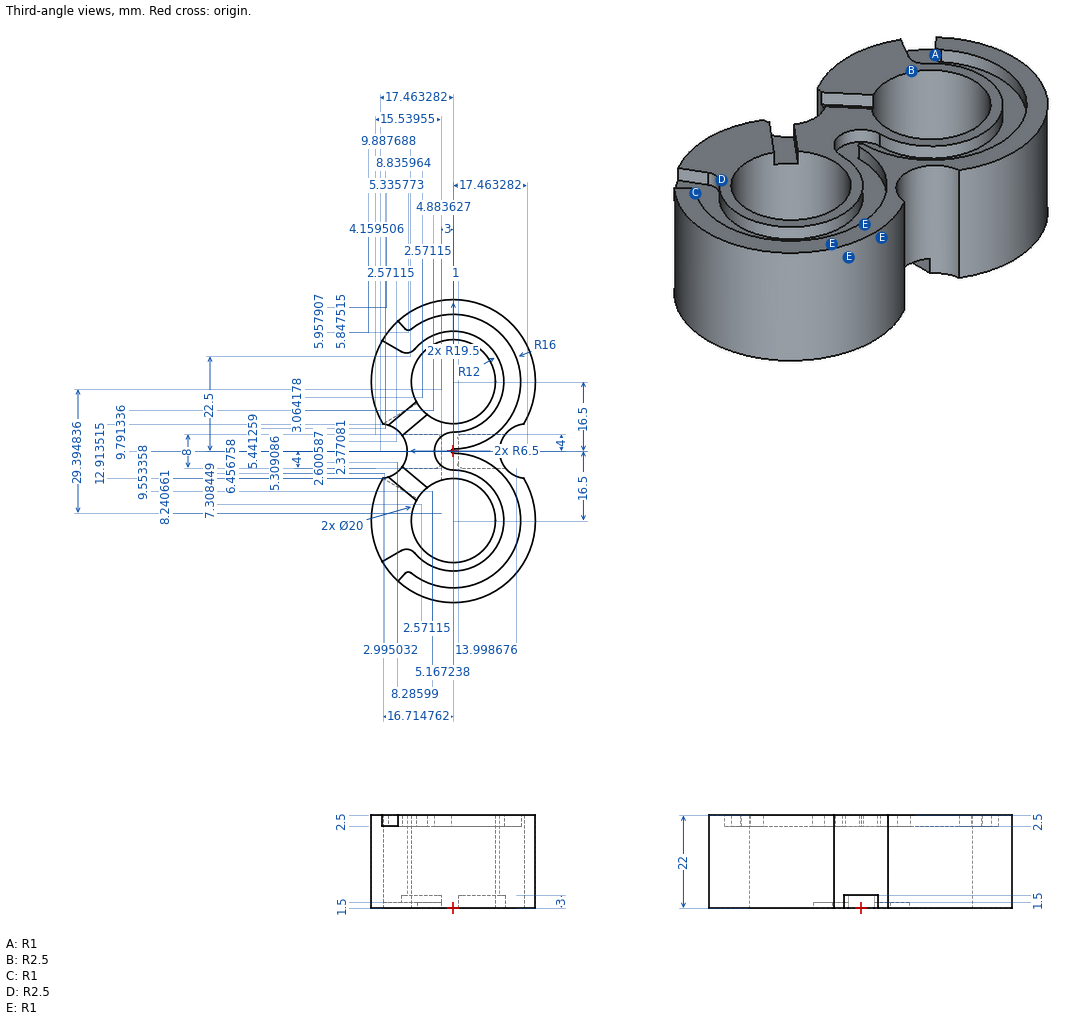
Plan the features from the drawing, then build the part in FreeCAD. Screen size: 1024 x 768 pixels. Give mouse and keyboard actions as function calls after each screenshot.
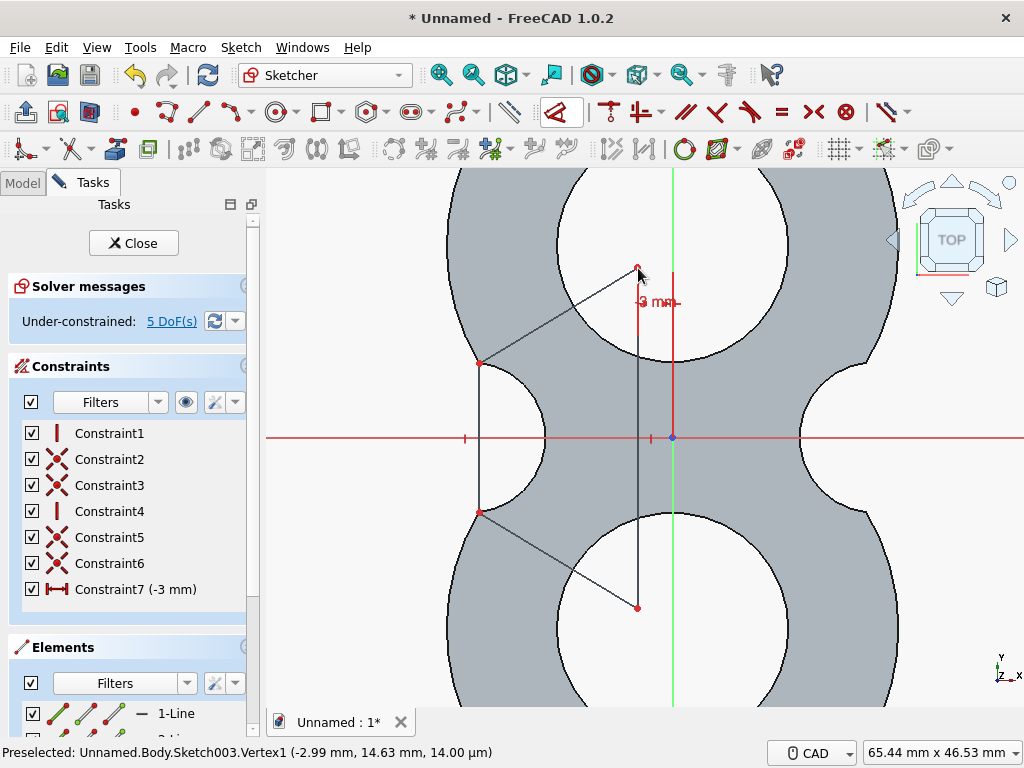
click(638, 370)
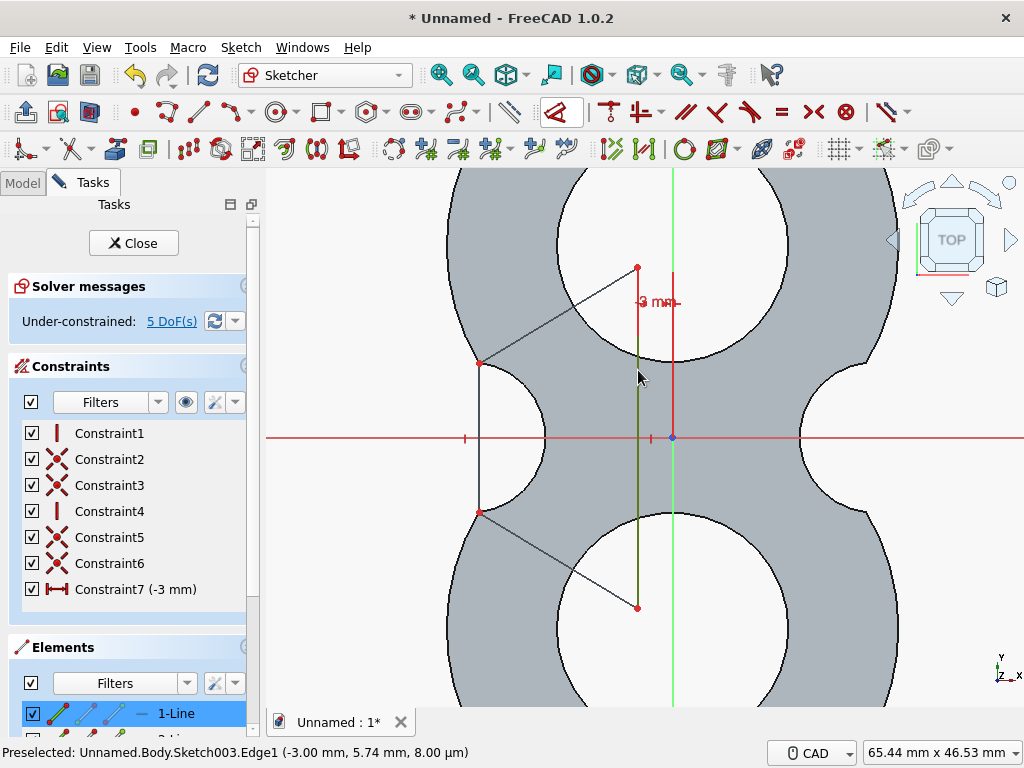
key(i)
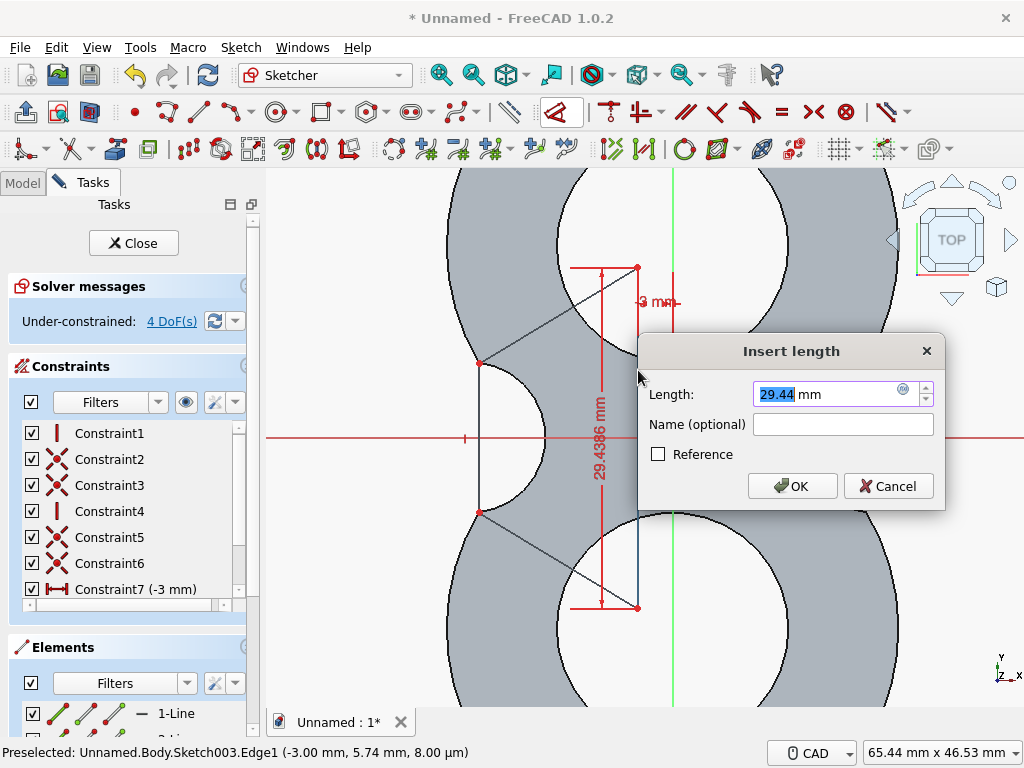
text(29.394836)
key(Return)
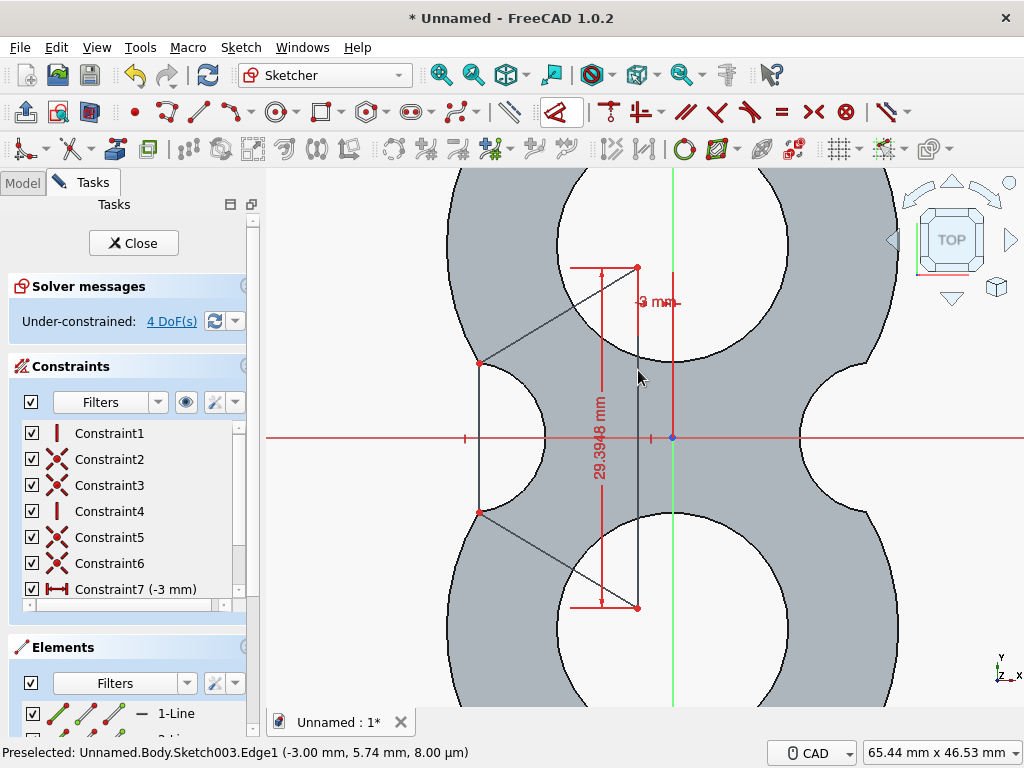
click(479, 468)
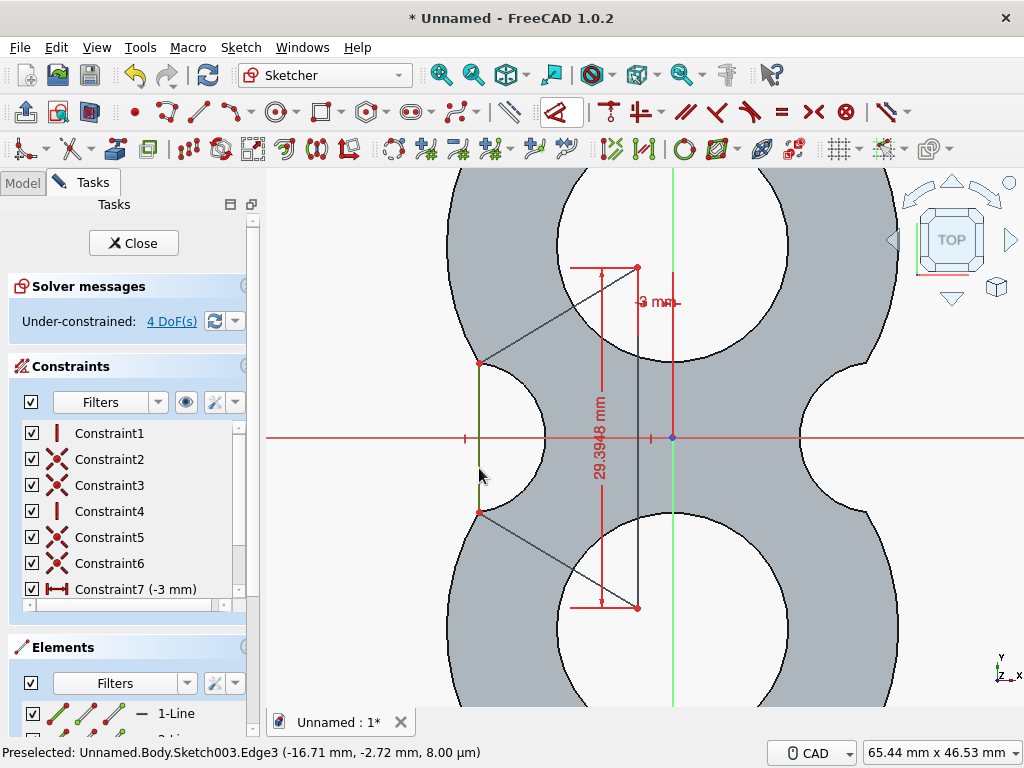
click(578, 112)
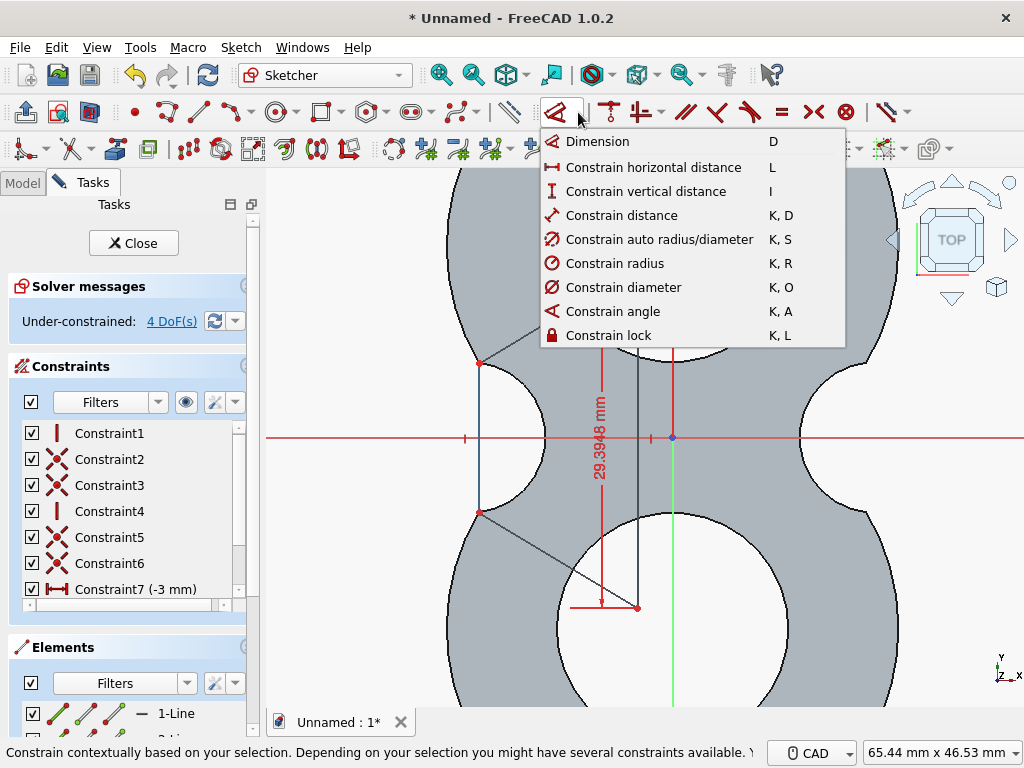
click(693, 191)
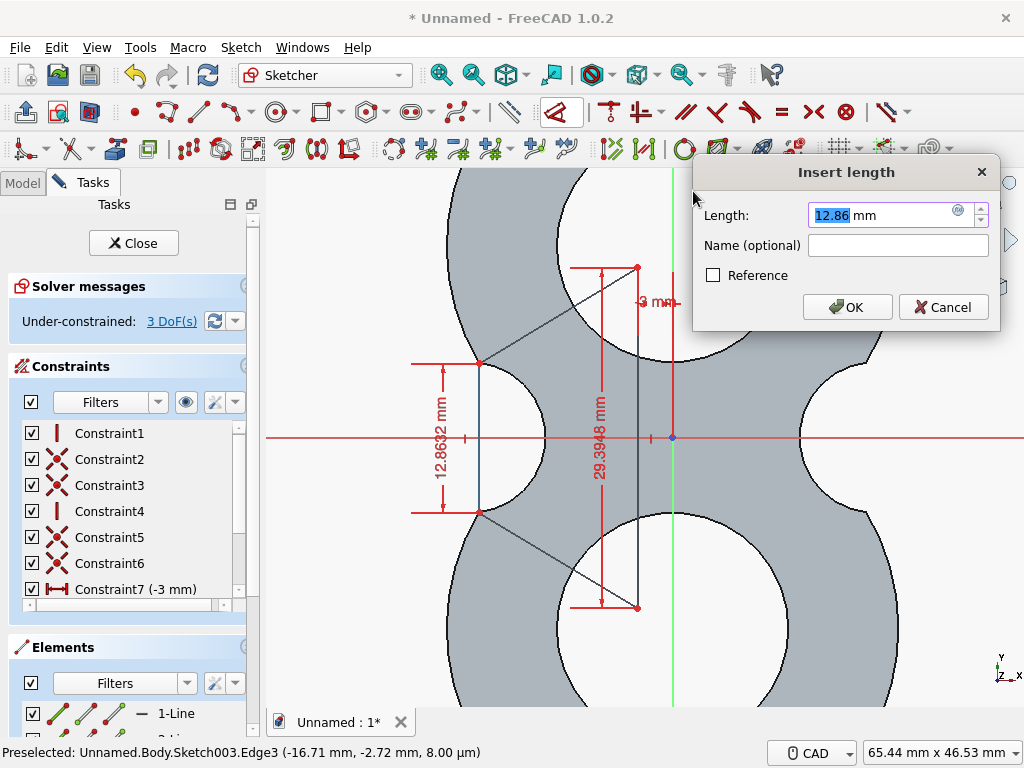
text(12.913515)
key(Return)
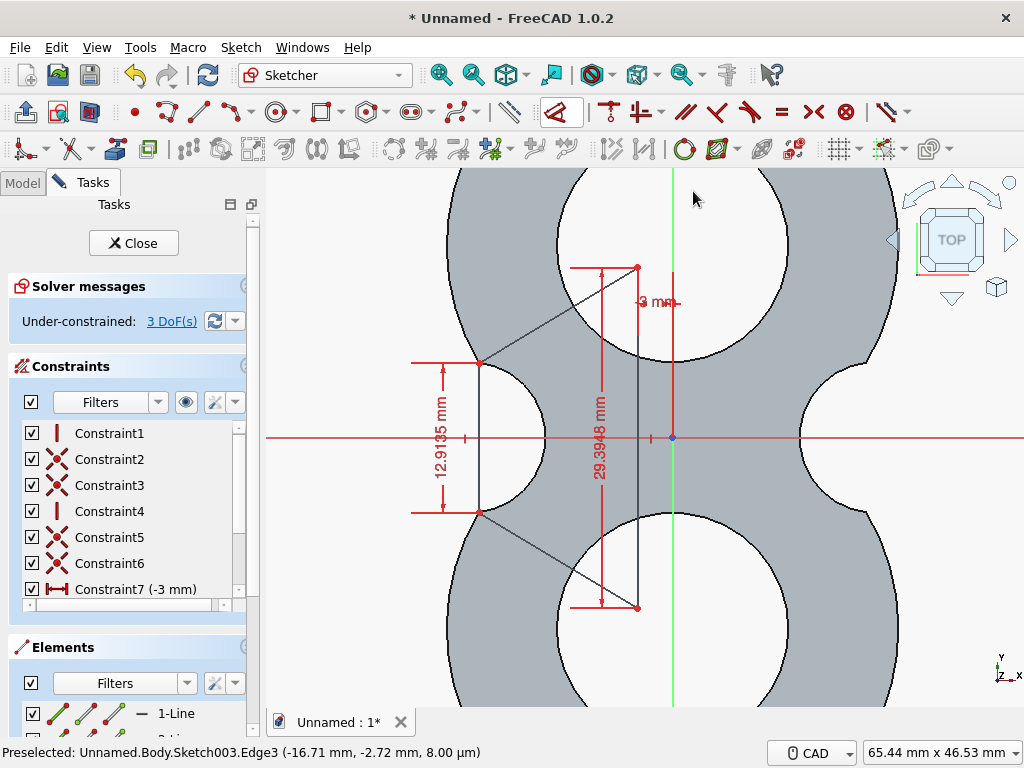
click(479, 513)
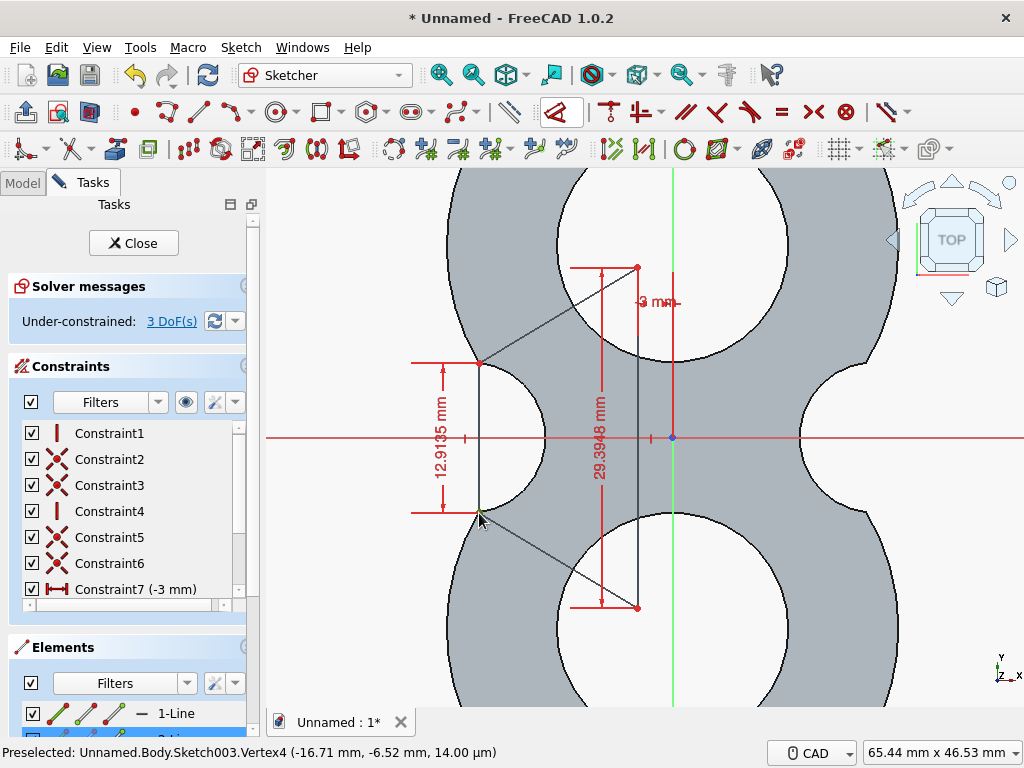
key(i)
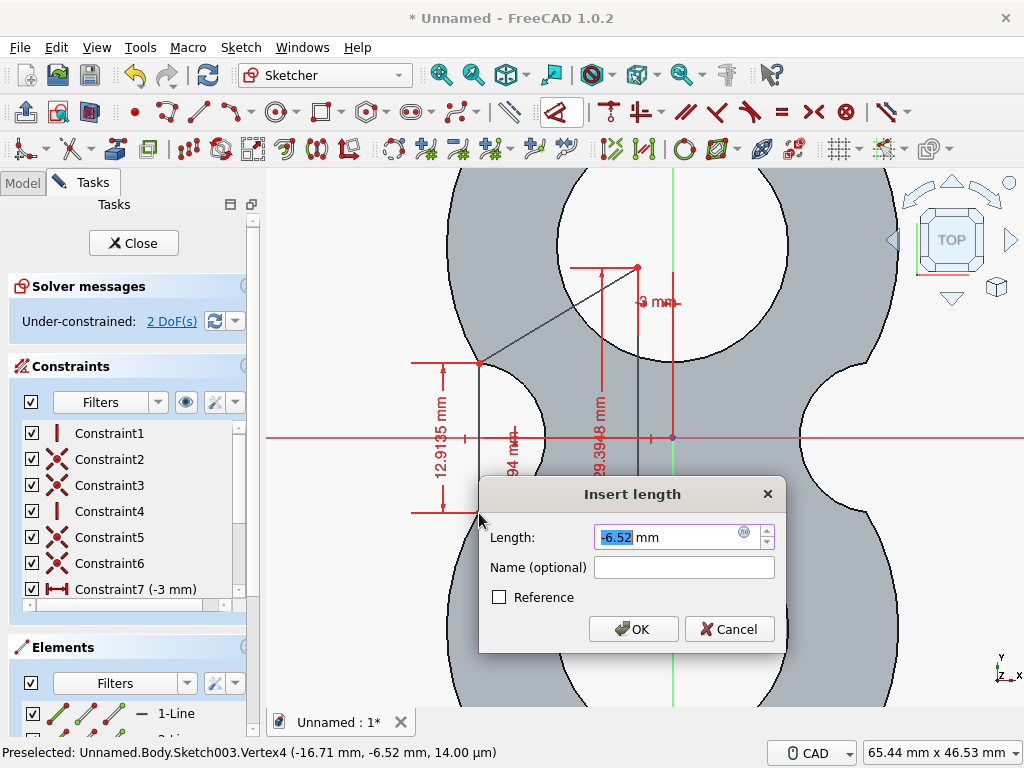
text(-6.456758)
key(Return)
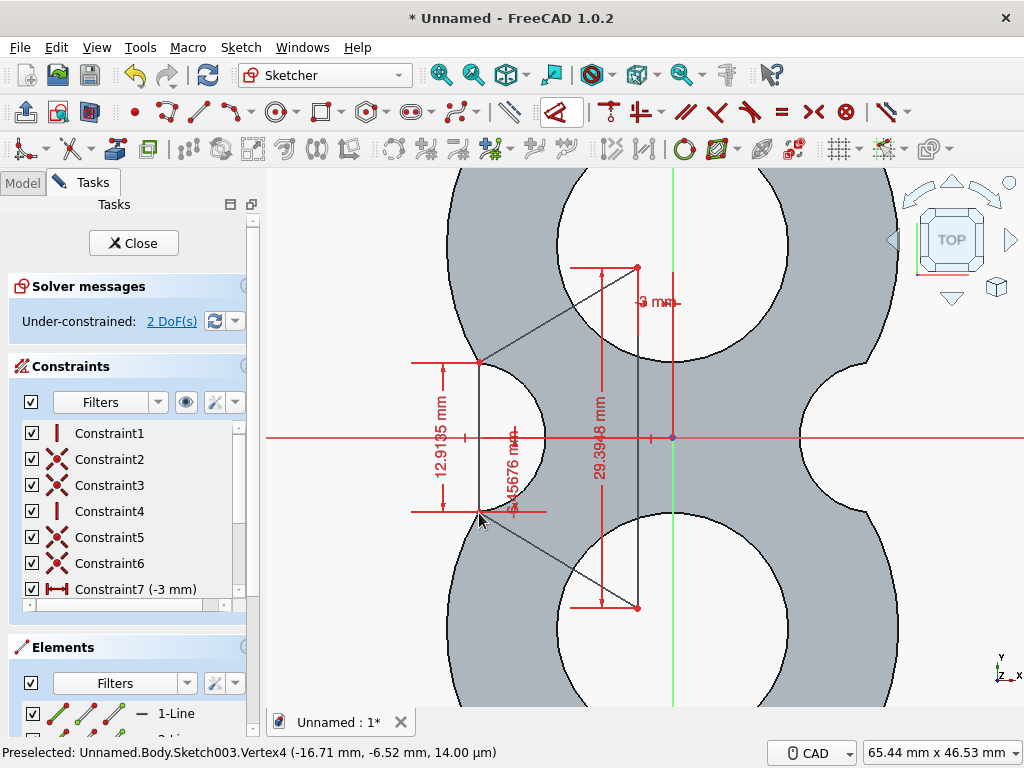
click(590, 580)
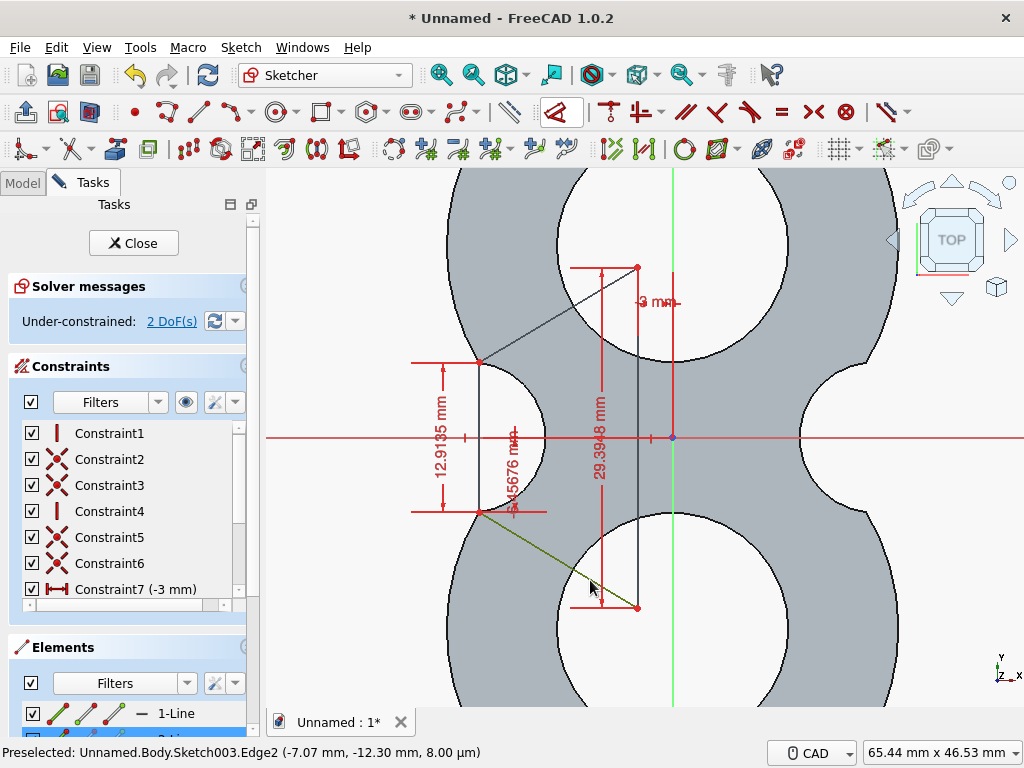
key(i)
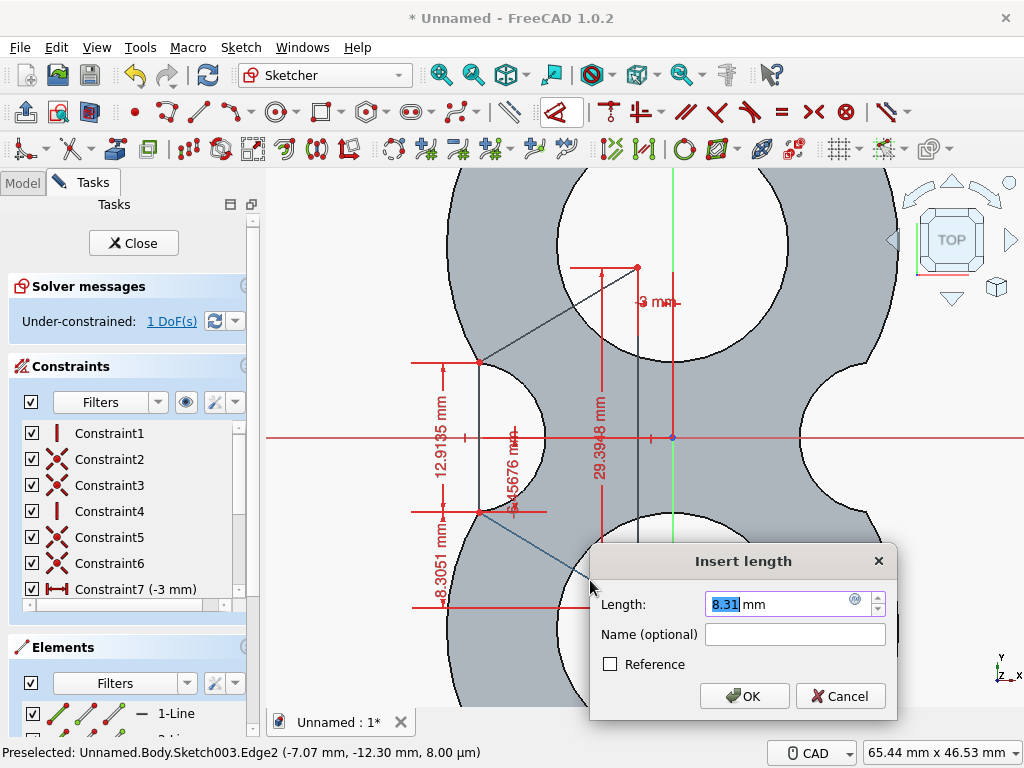
text(8.240661)
key(Return)